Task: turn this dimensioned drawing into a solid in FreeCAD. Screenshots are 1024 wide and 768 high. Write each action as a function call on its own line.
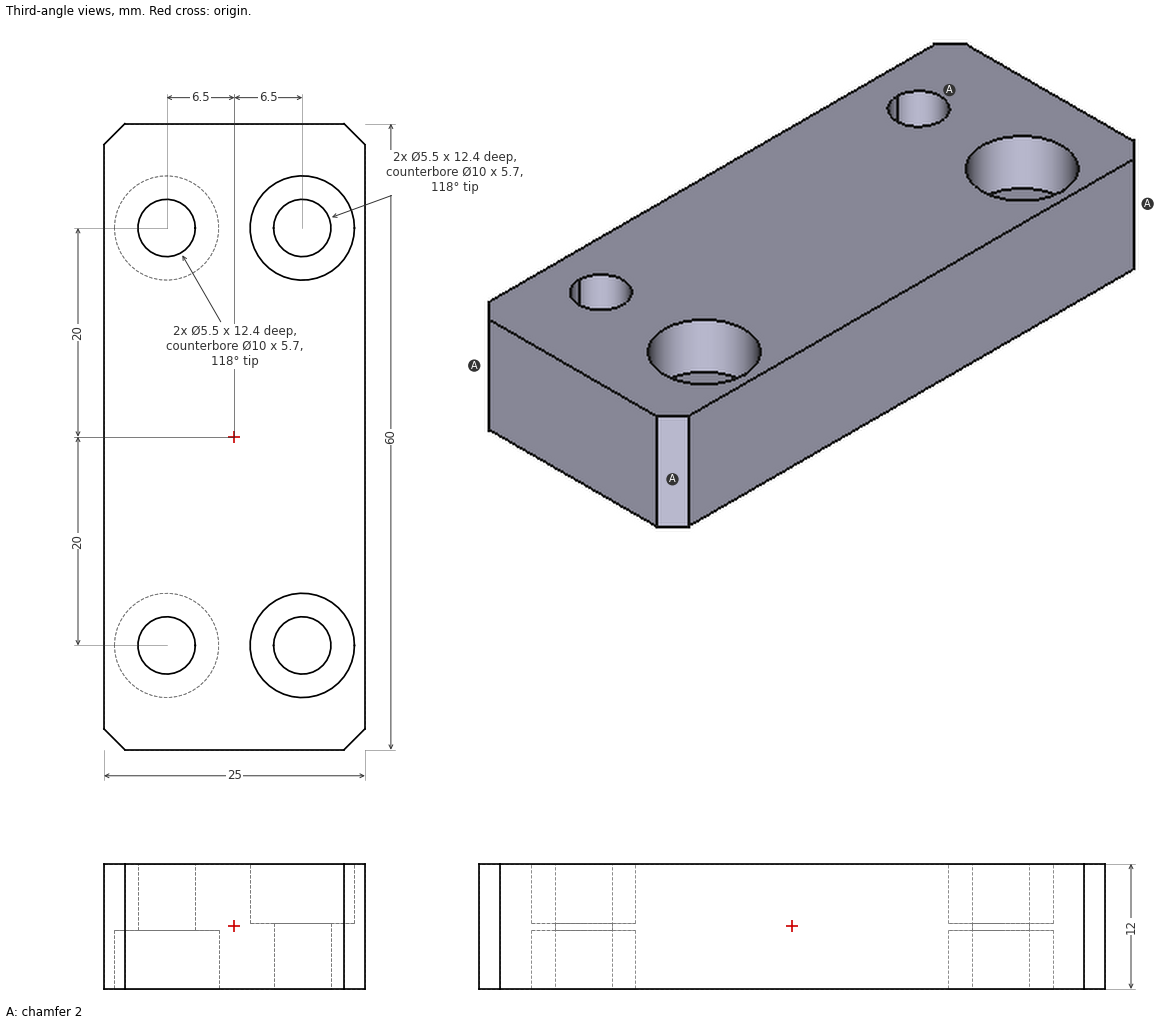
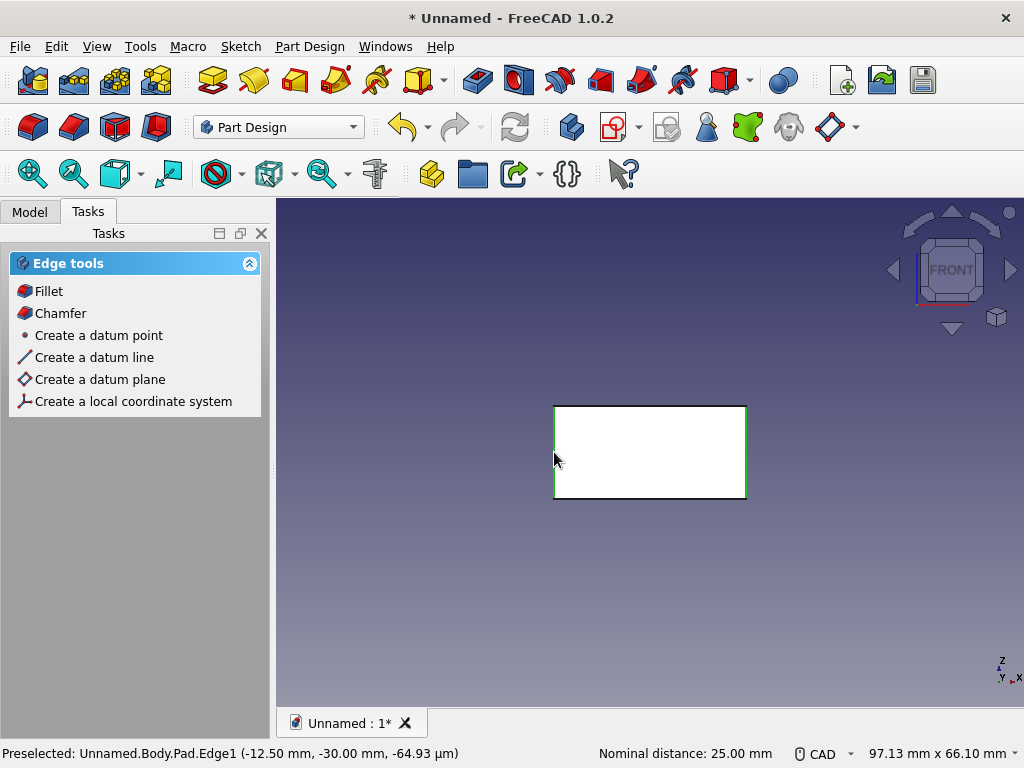
key(3)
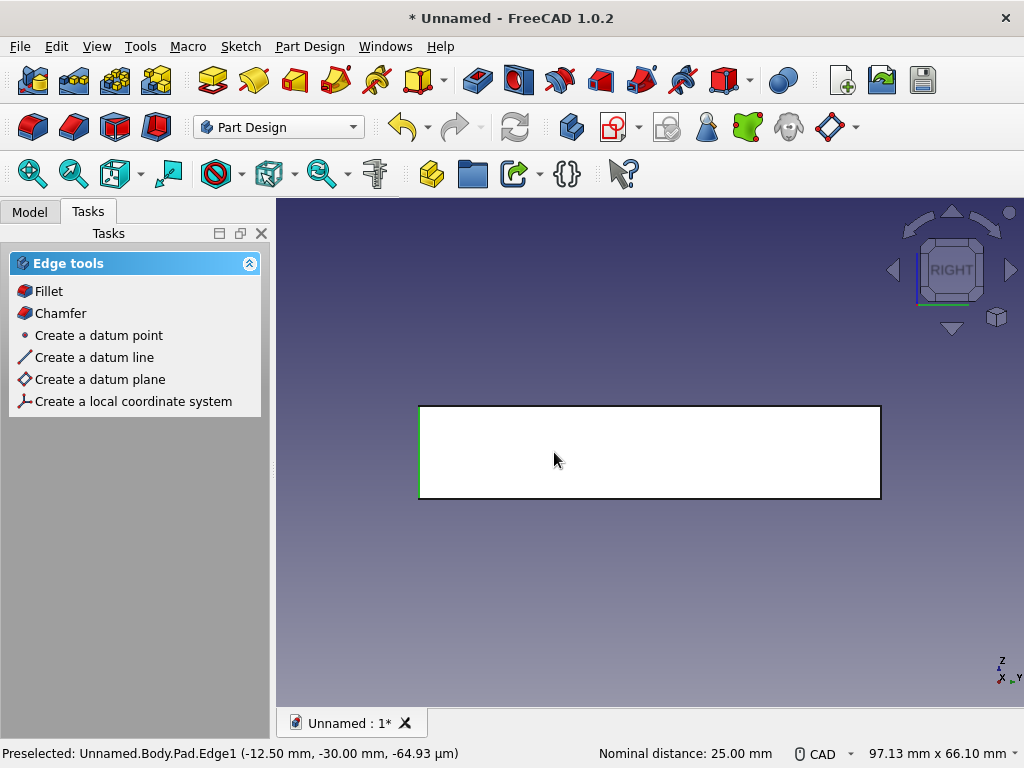
click(881, 451, ctrl)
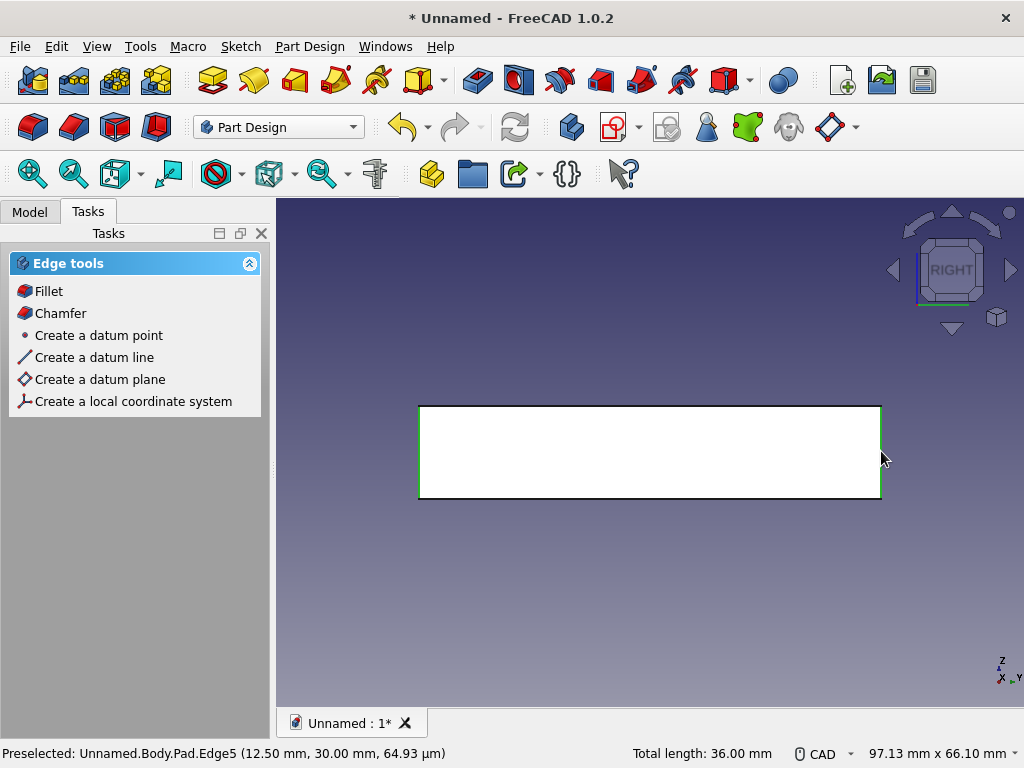
key(5)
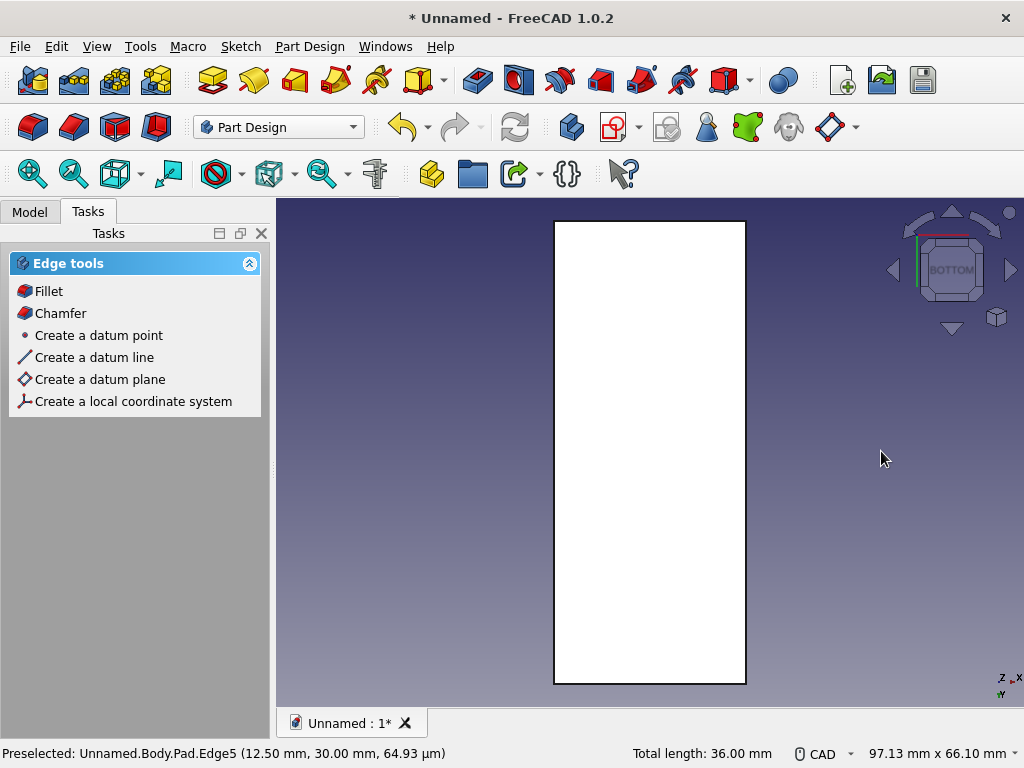
key(4)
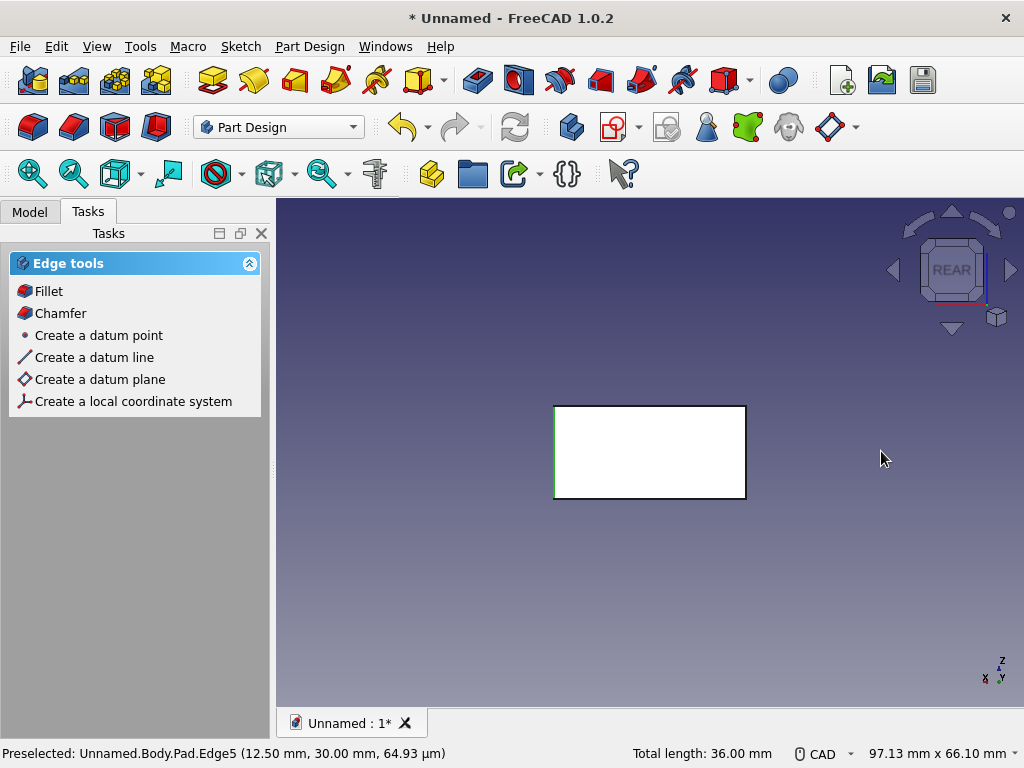
click(33, 174)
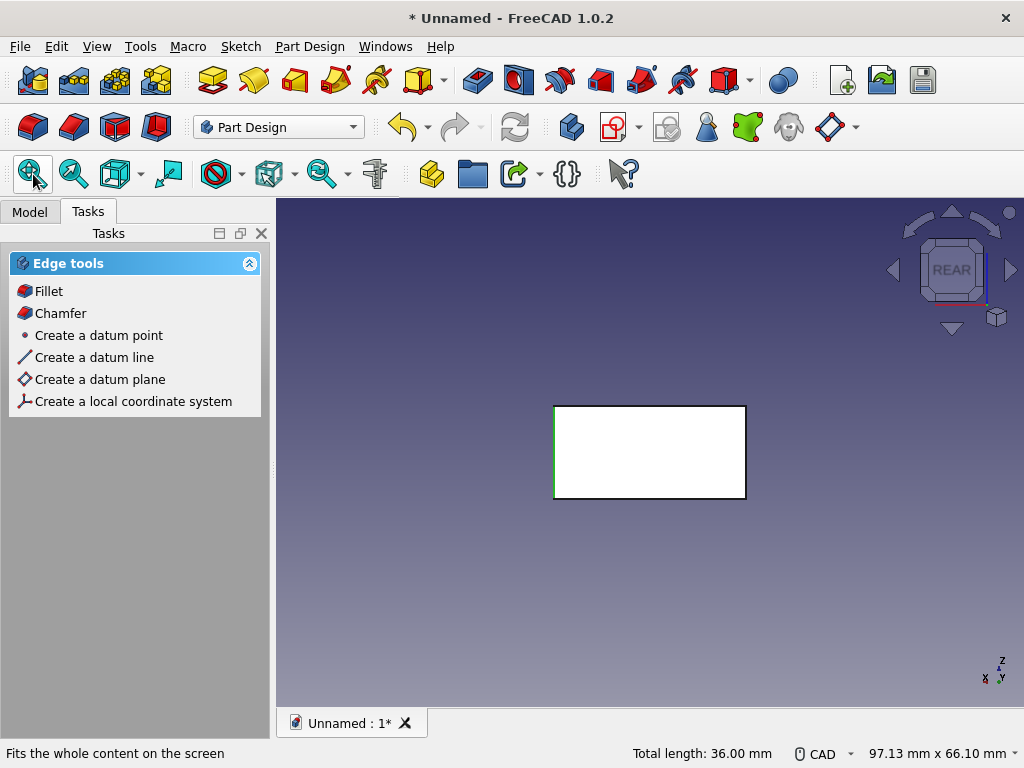
click(746, 452, ctrl)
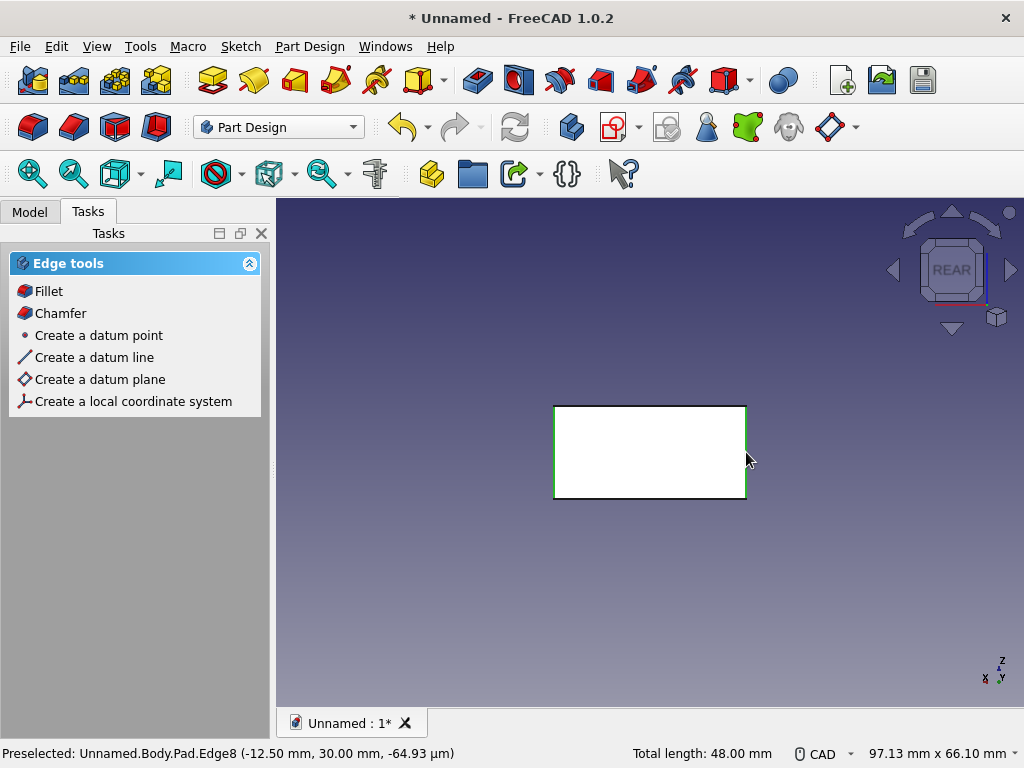
click(74, 128)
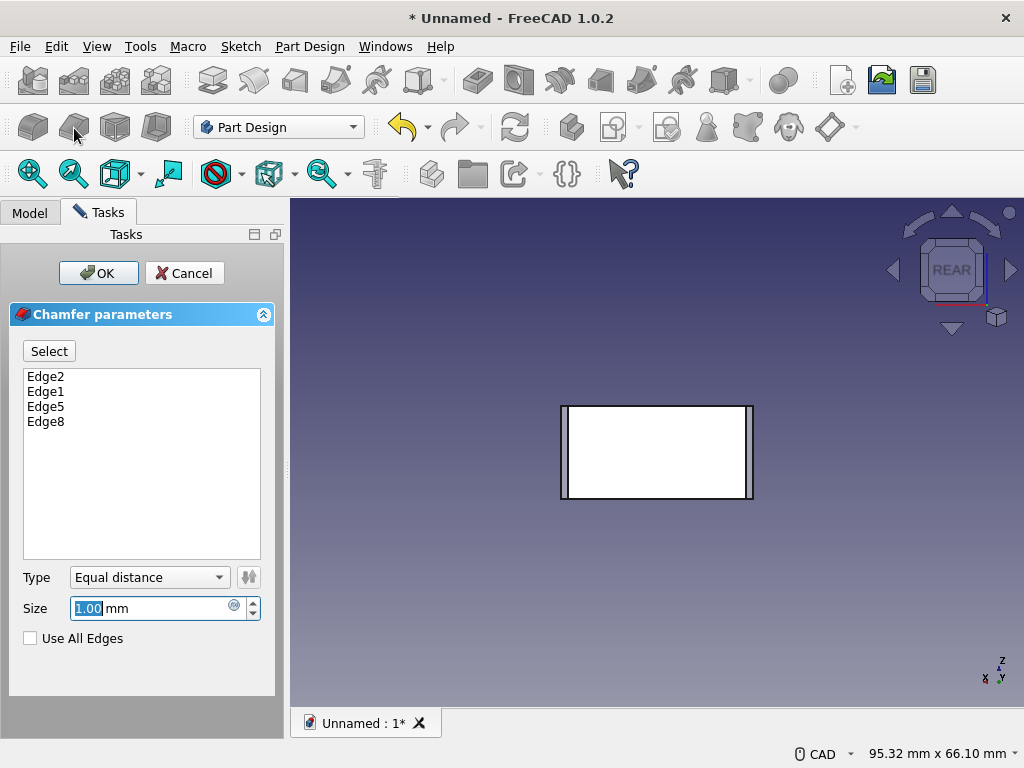
text(2)
key(Tab)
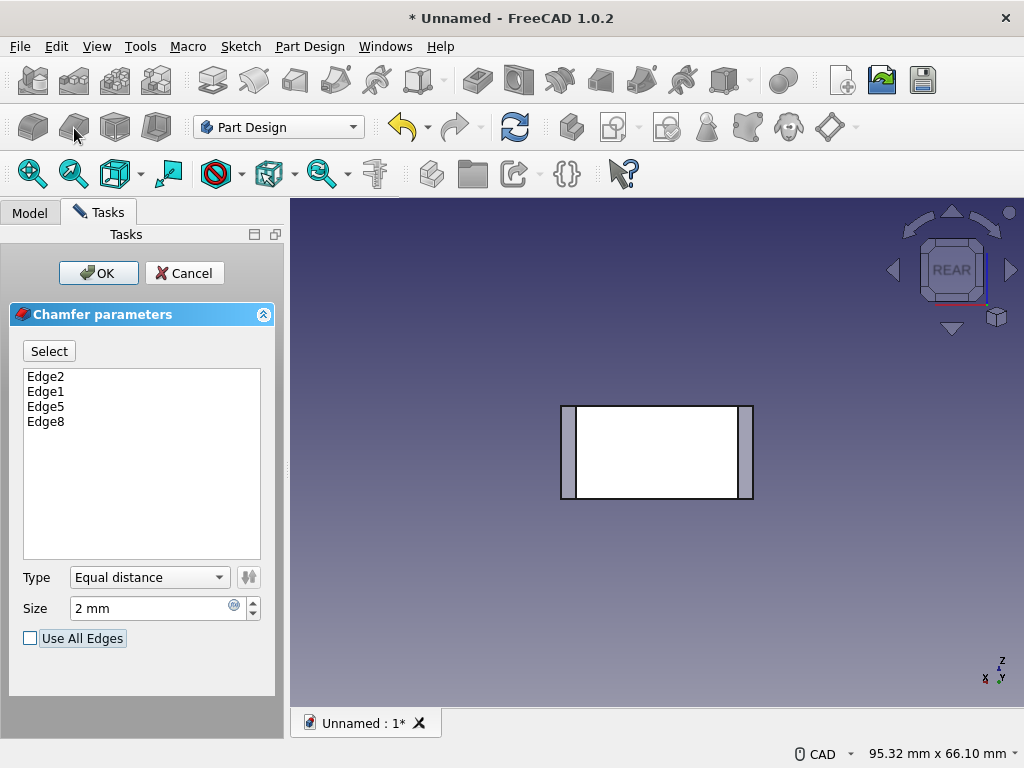
click(99, 273)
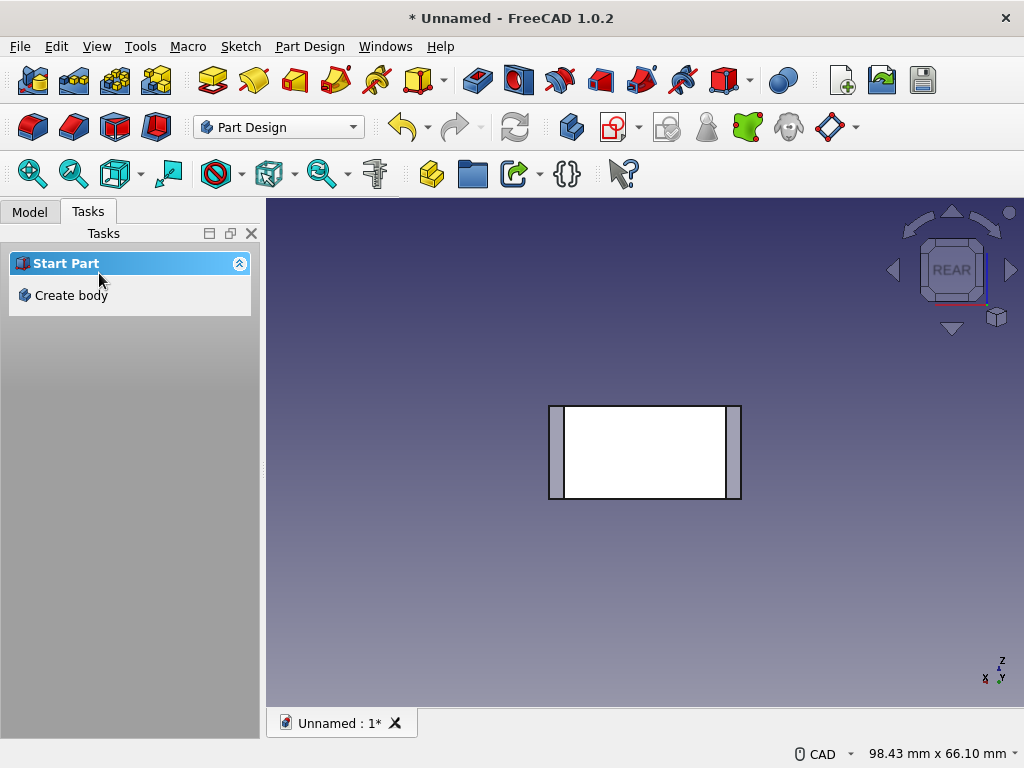
click(33, 174)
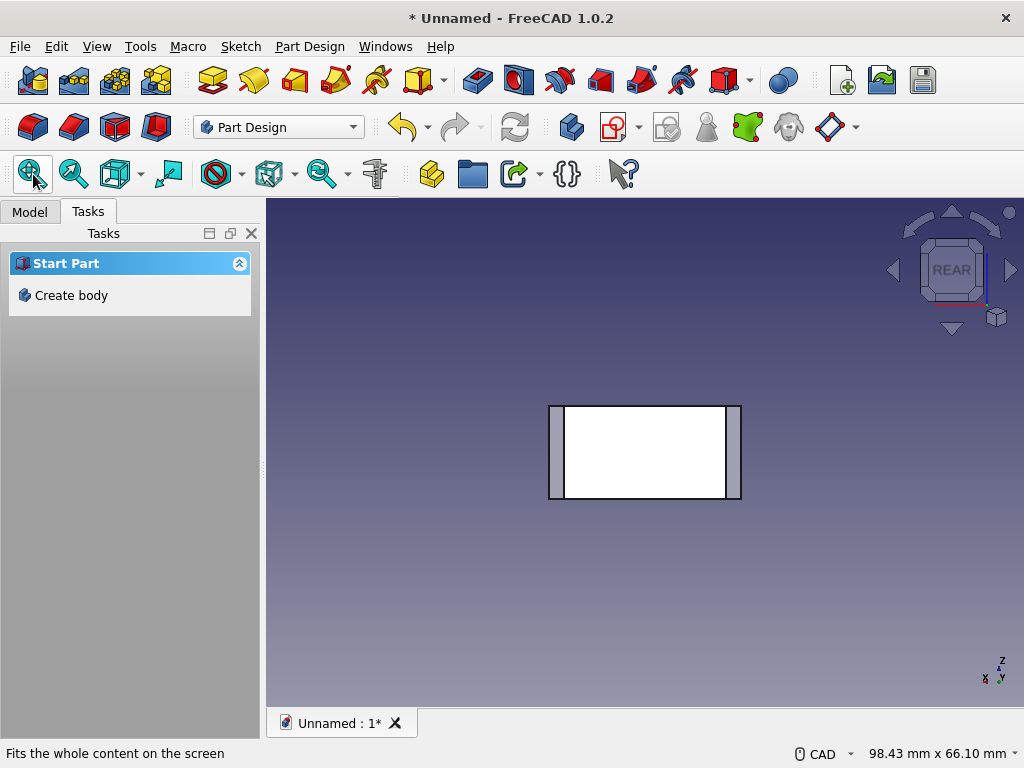
key(5)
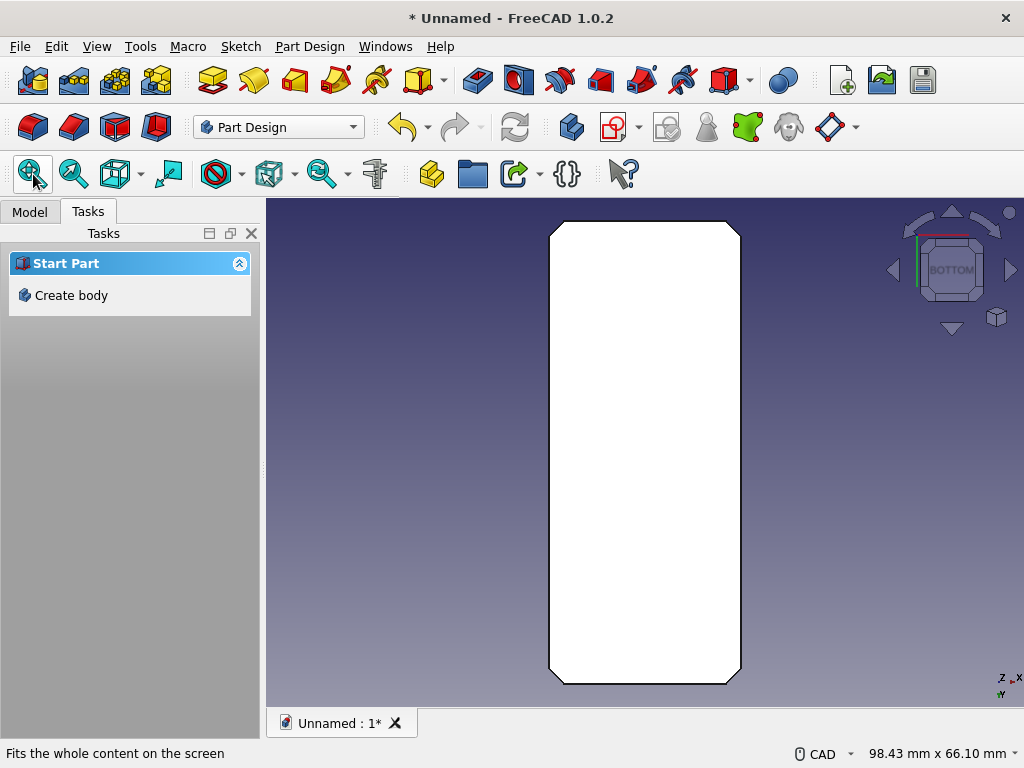
click(645, 584)